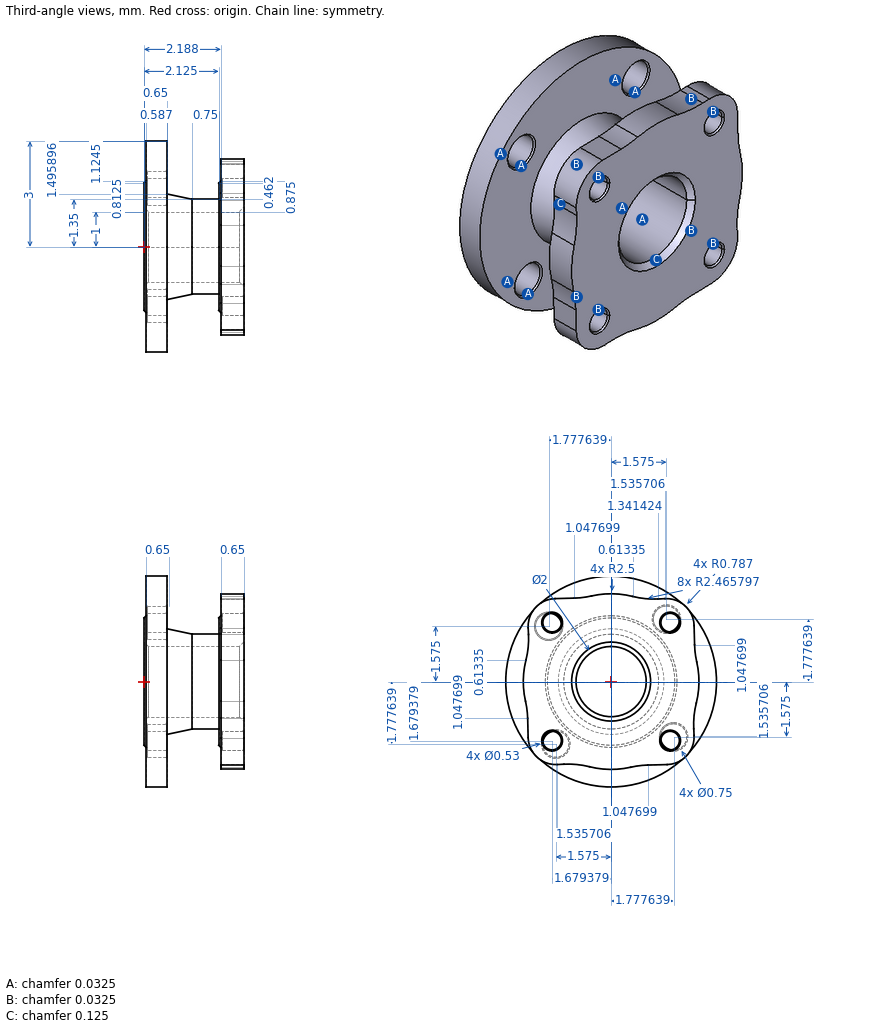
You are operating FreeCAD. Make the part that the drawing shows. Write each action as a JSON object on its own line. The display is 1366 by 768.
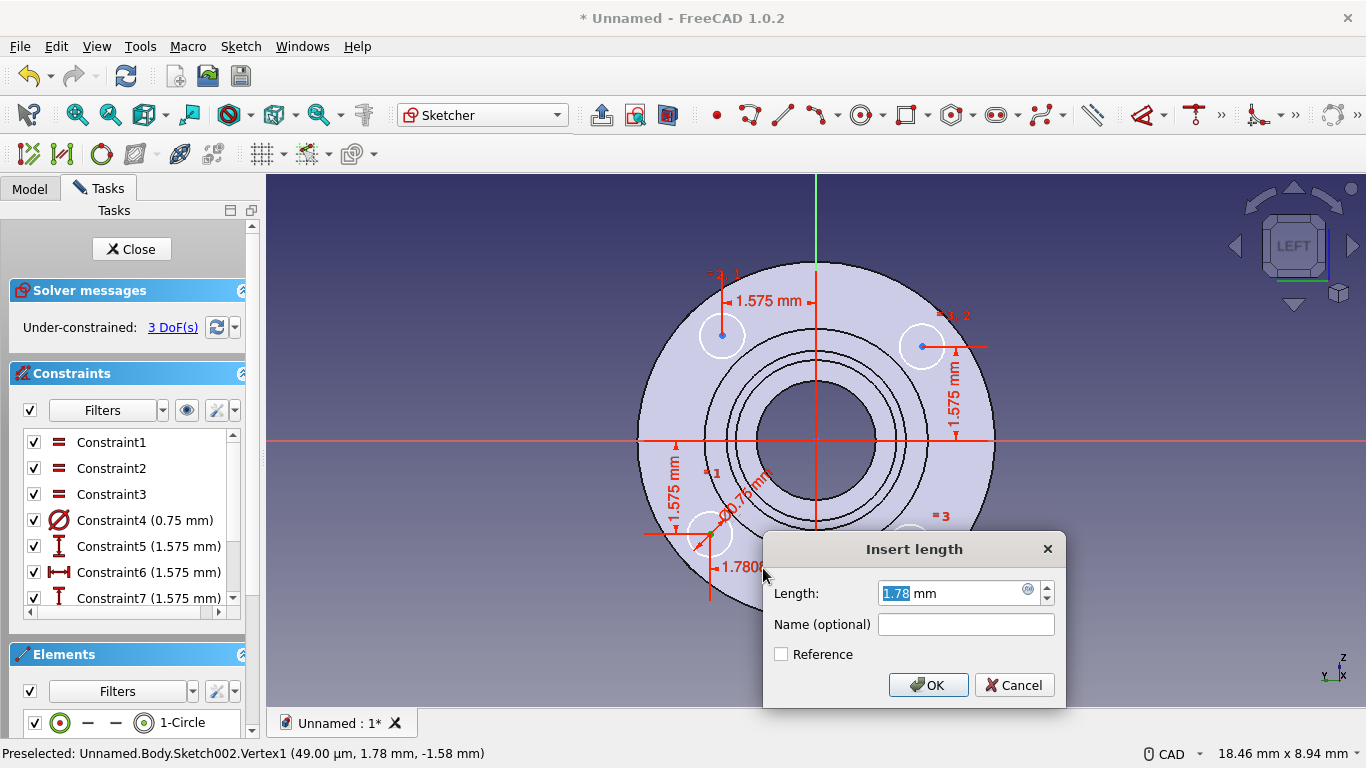
{"action": "type", "text": "1.777639"}
{"action": "key", "text": "Return"}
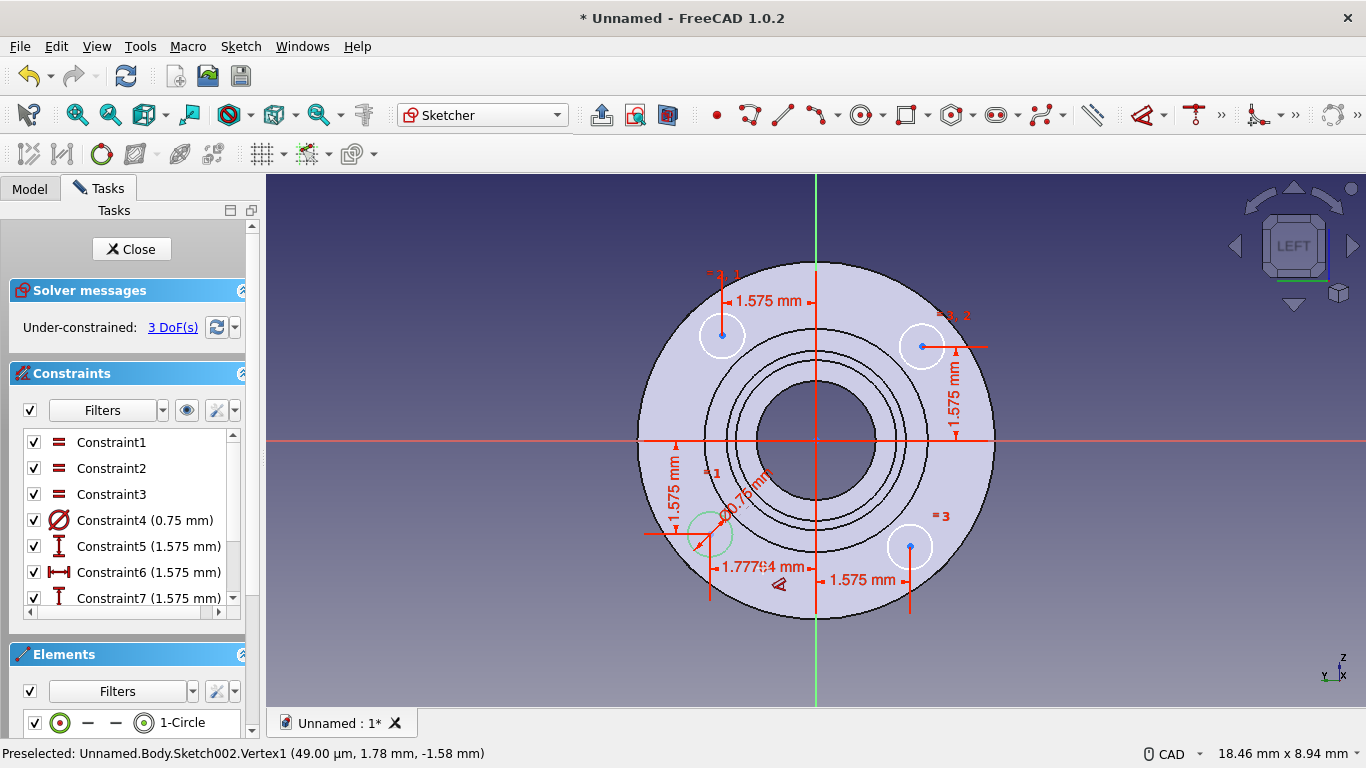
{"action": "left_click", "coordinate": [722, 336]}
{"action": "left_click", "coordinate": [688, 388]}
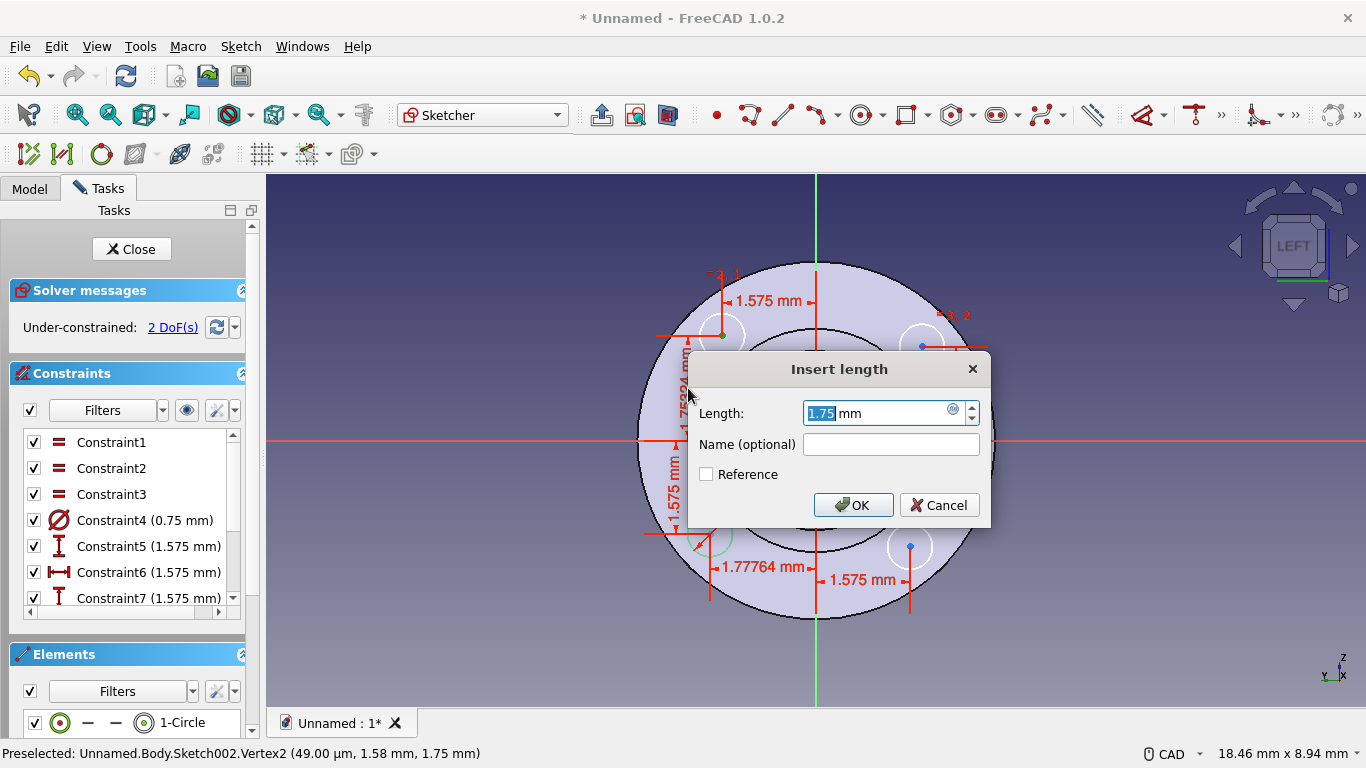
{"action": "type", "text": "1.777639"}
{"action": "key", "text": "Return"}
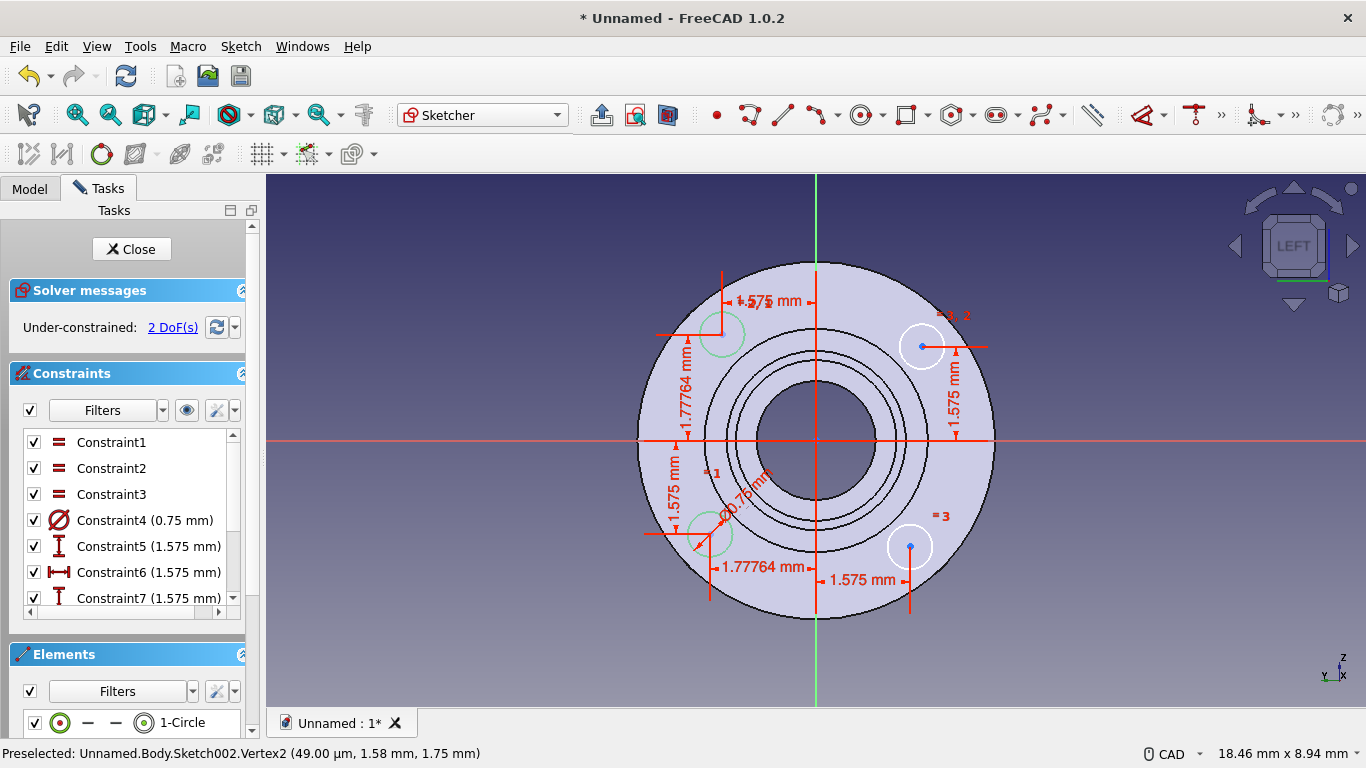
{"action": "left_click", "coordinate": [922, 347]}
{"action": "left_click", "coordinate": [869, 313]}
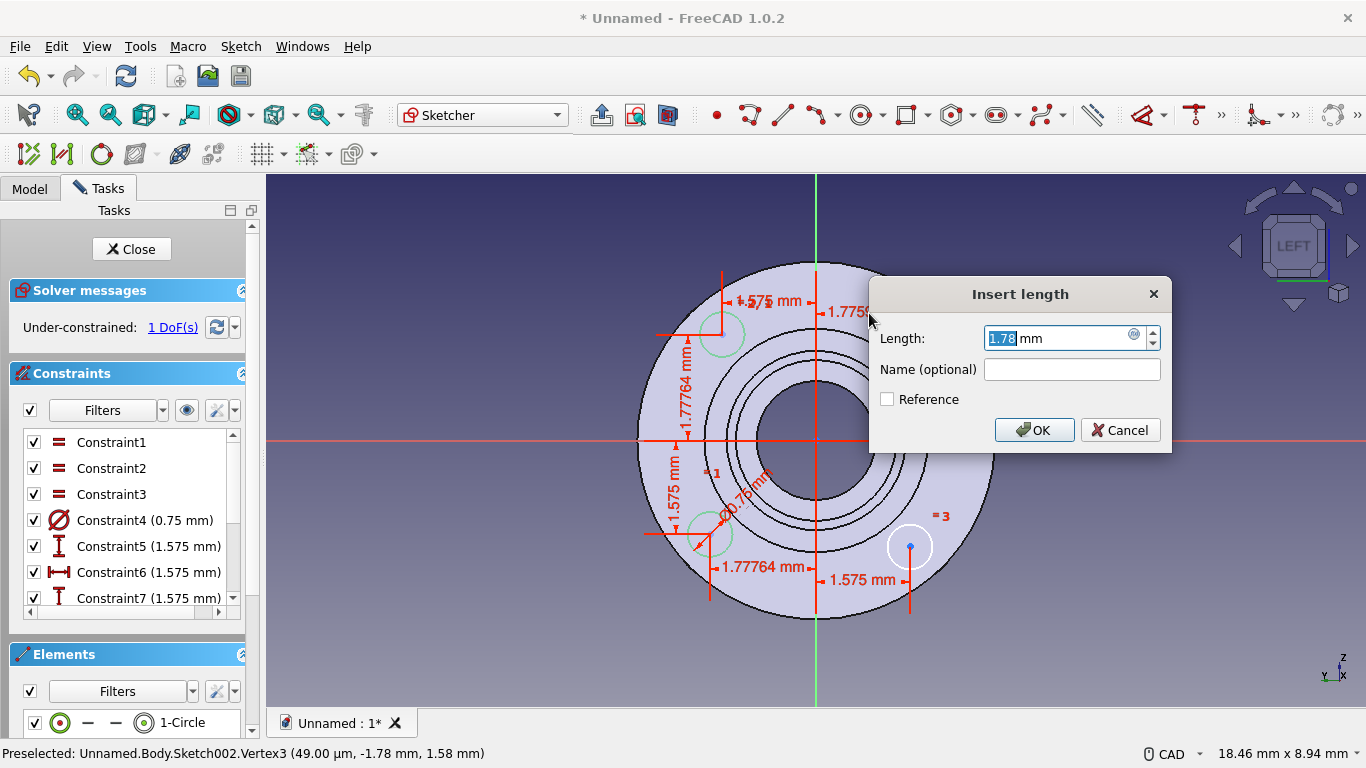
{"action": "type", "text": "1.777639"}
{"action": "key", "text": "Return"}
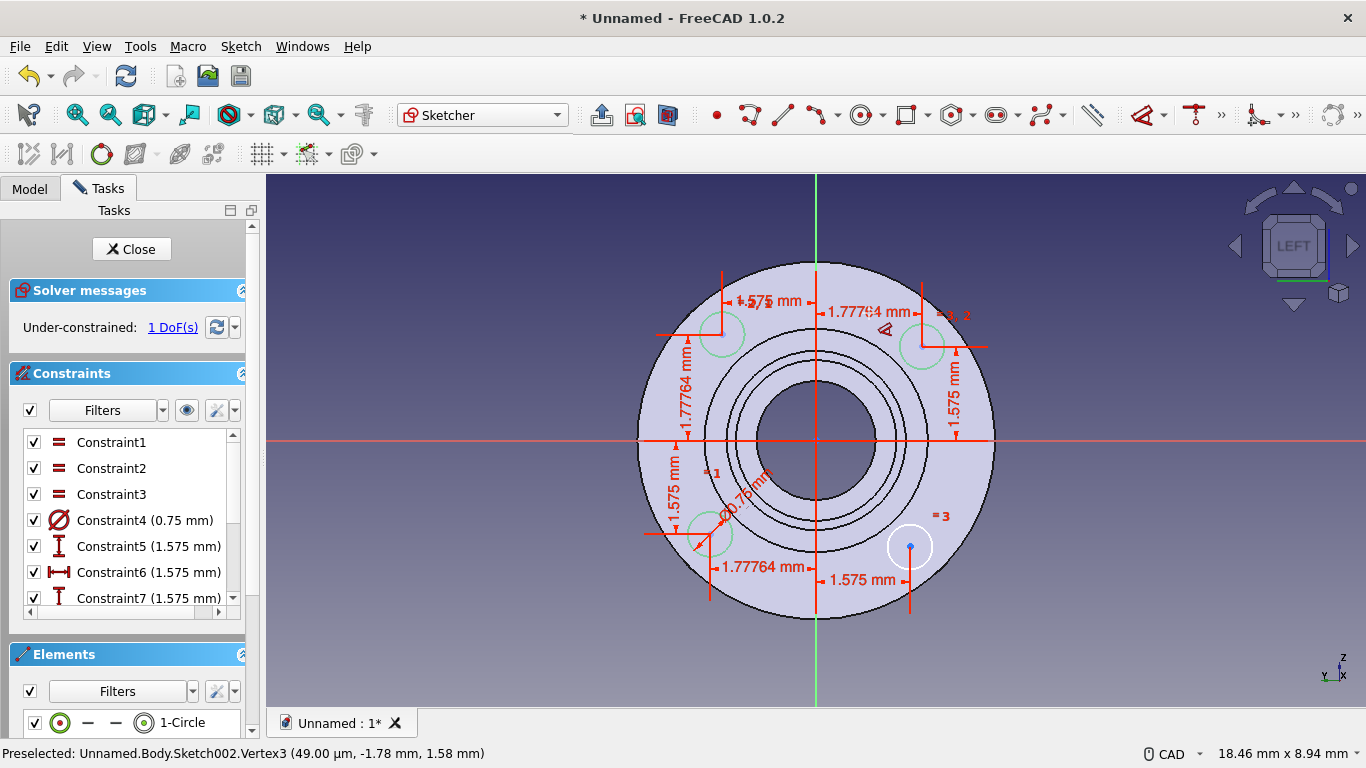
{"action": "left_click", "coordinate": [910, 547]}
{"action": "left_click", "coordinate": [944, 494]}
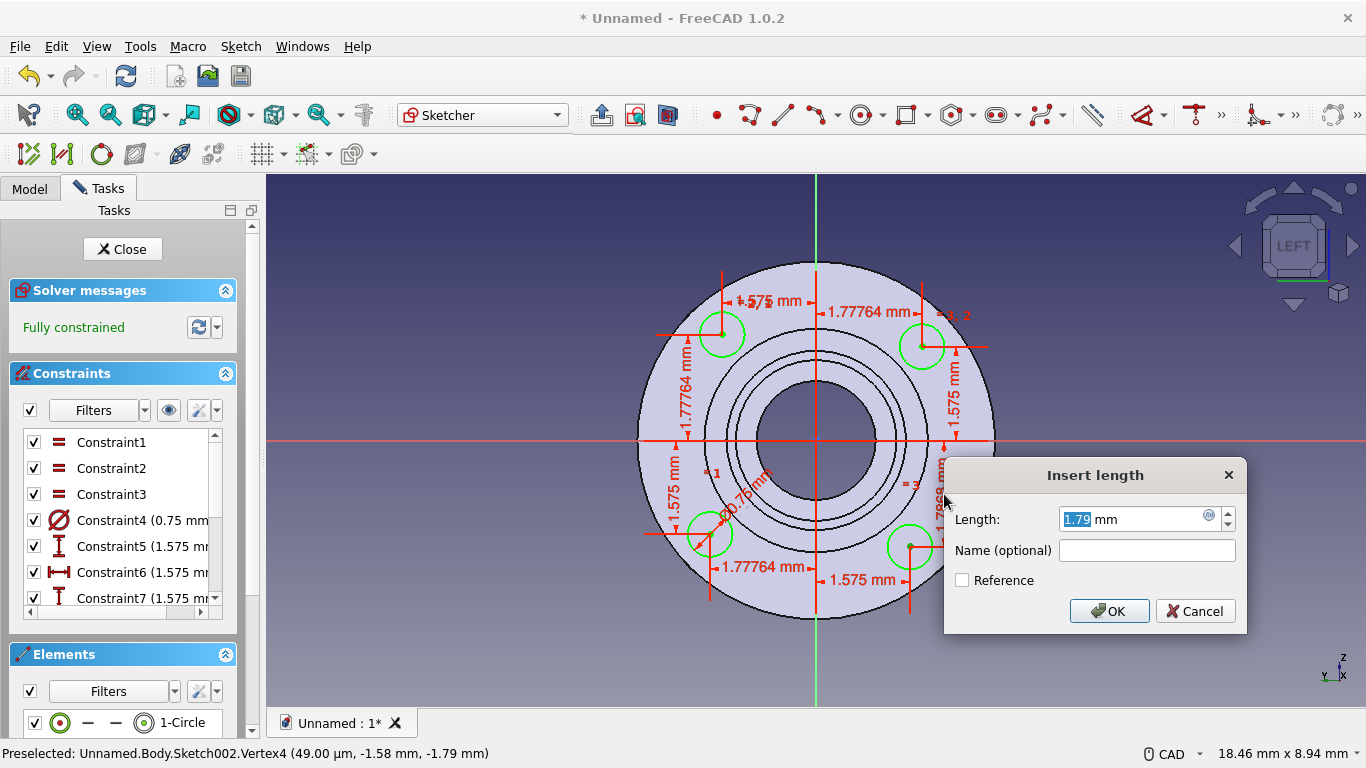
{"action": "type", "text": "1.777639"}
{"action": "key", "text": "Return"}
{"action": "key", "text": "Escape"}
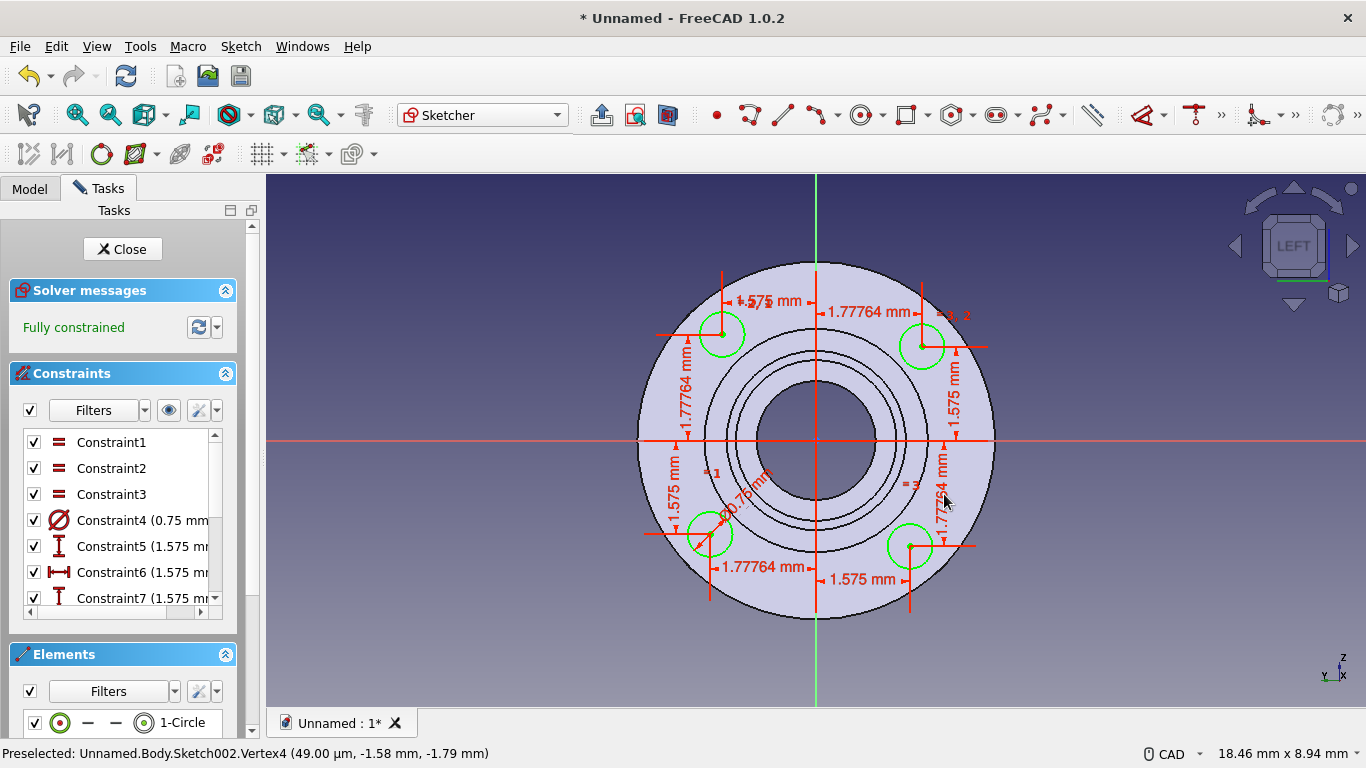
{"action": "left_click", "coordinate": [123, 249]}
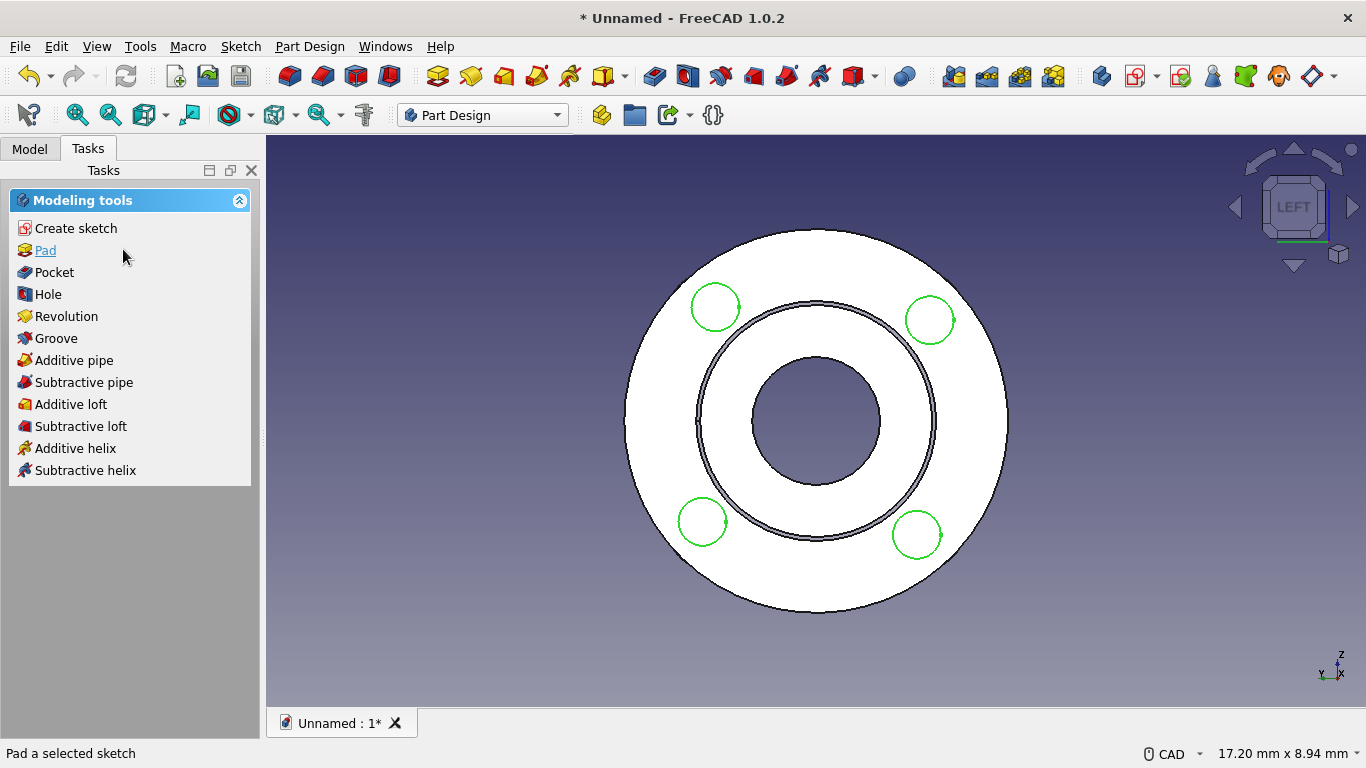
{"action": "left_click", "coordinate": [655, 76]}